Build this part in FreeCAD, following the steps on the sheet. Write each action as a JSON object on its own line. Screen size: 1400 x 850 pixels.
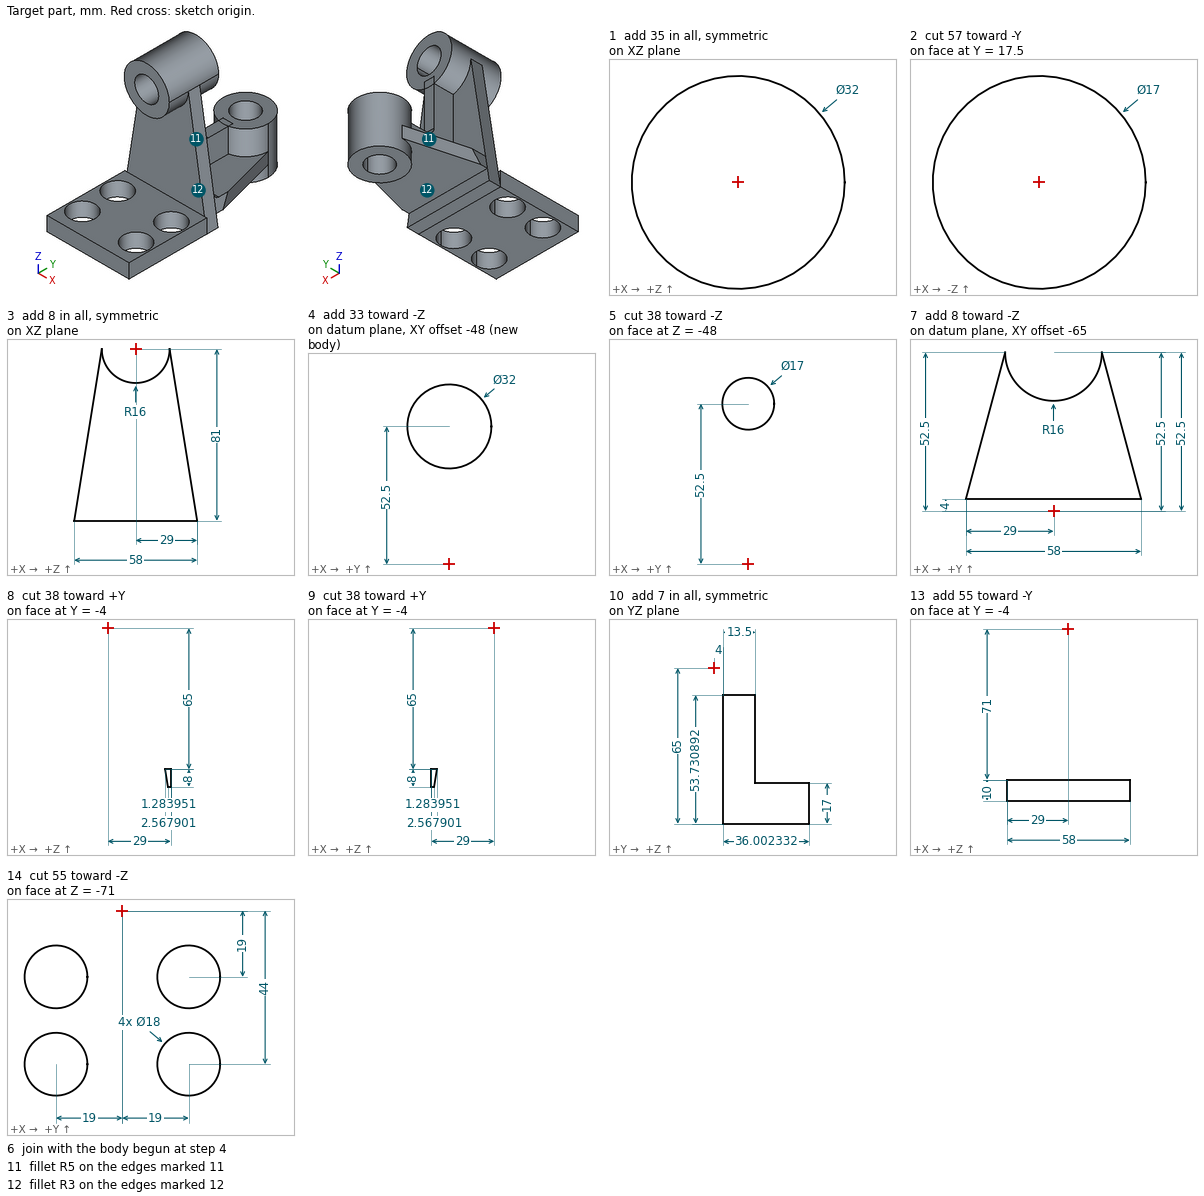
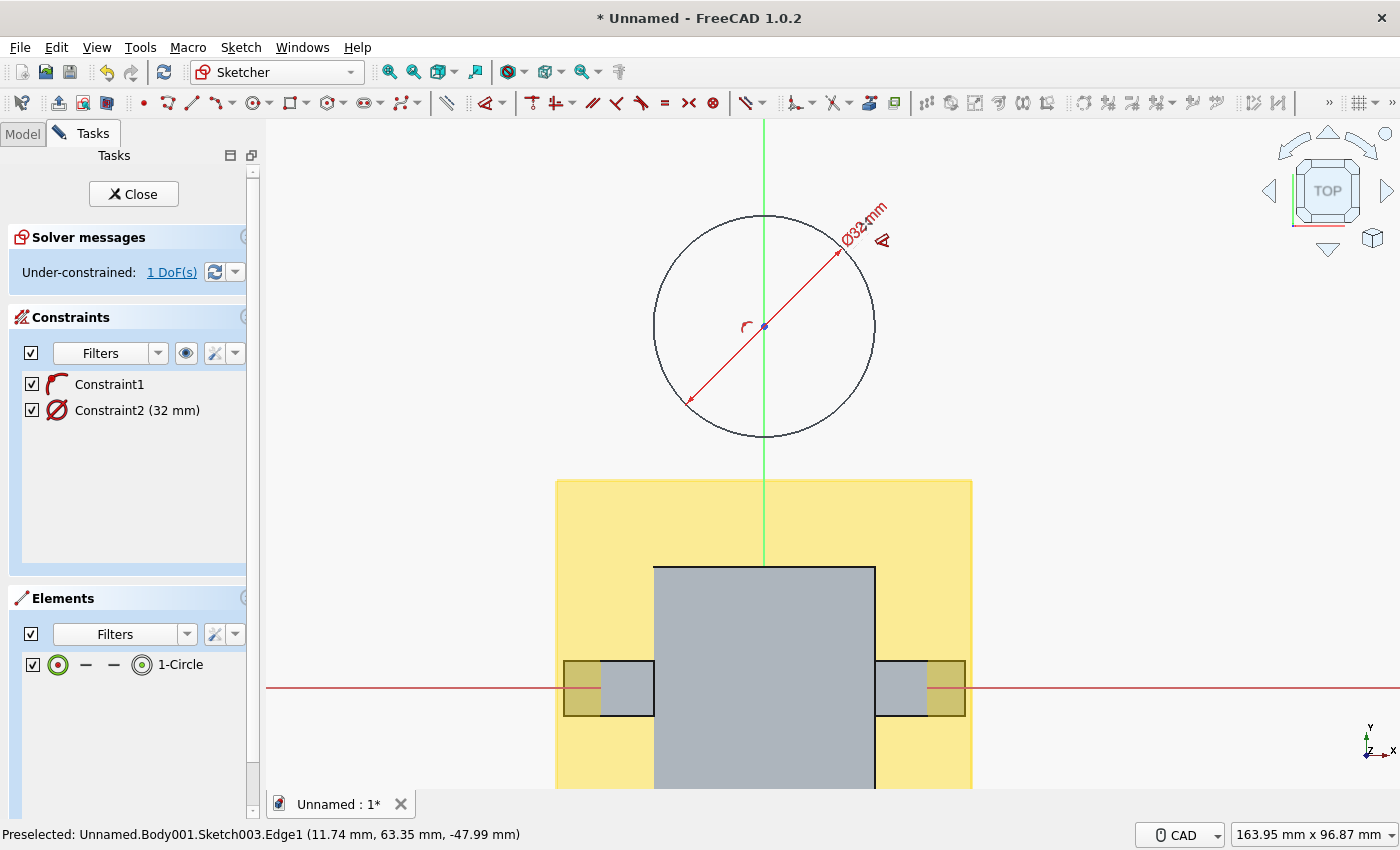
{"action": "left_click", "coordinate": [764, 326]}
{"action": "left_click", "coordinate": [798, 507]}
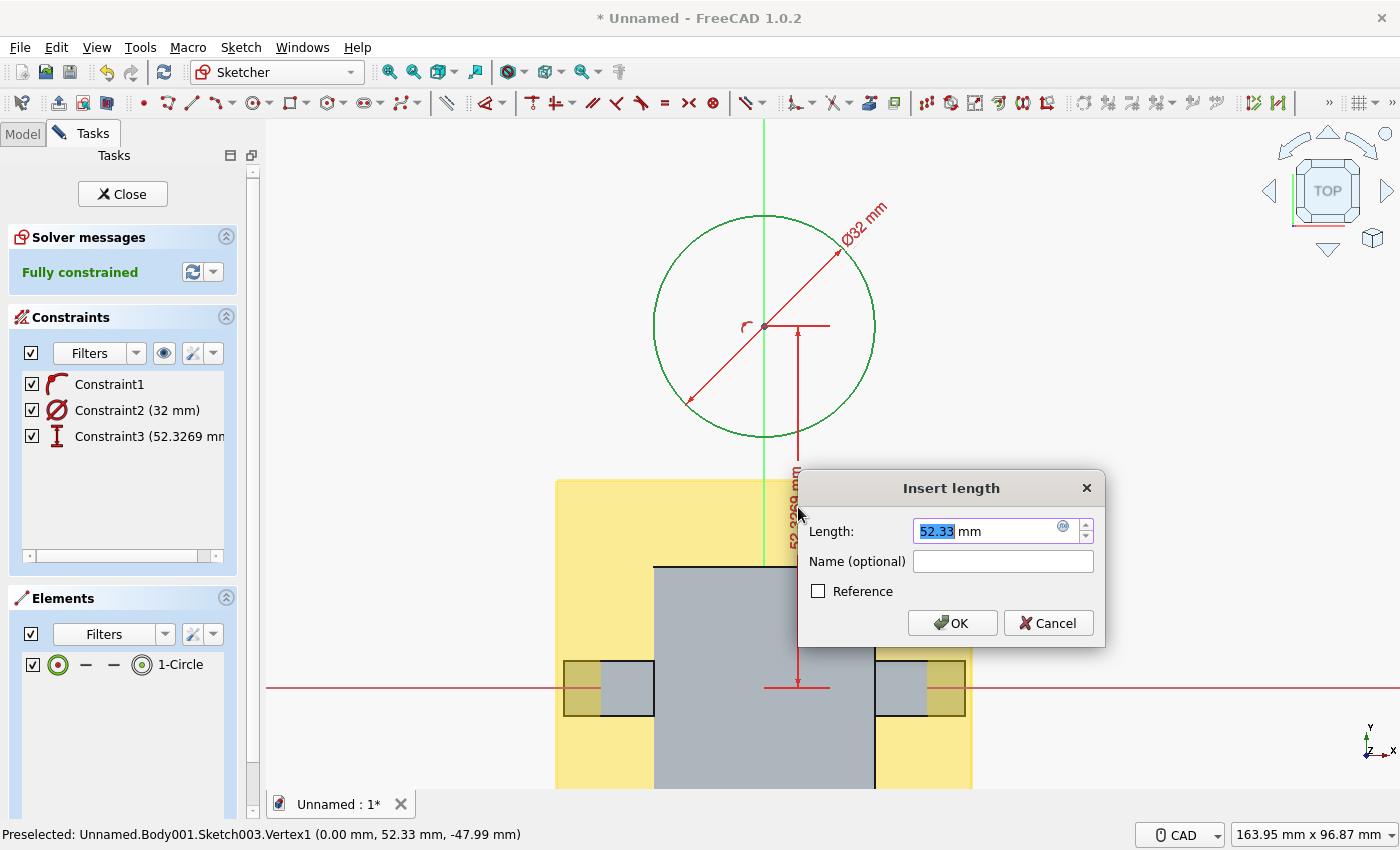
{"action": "type", "text": "52.5"}
{"action": "key", "text": "Return"}
{"action": "key", "text": "Escape"}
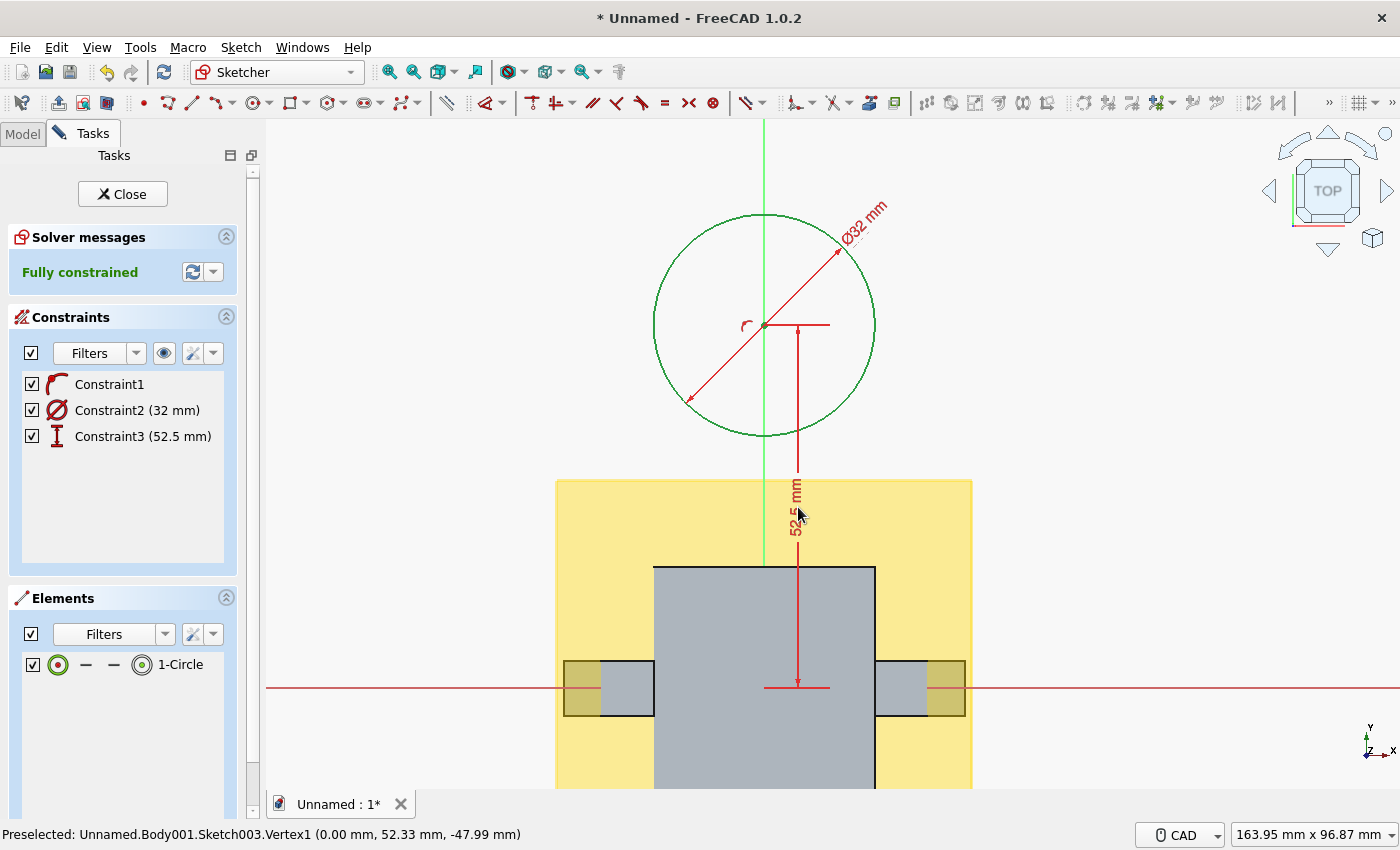
{"action": "left_click", "coordinate": [123, 194]}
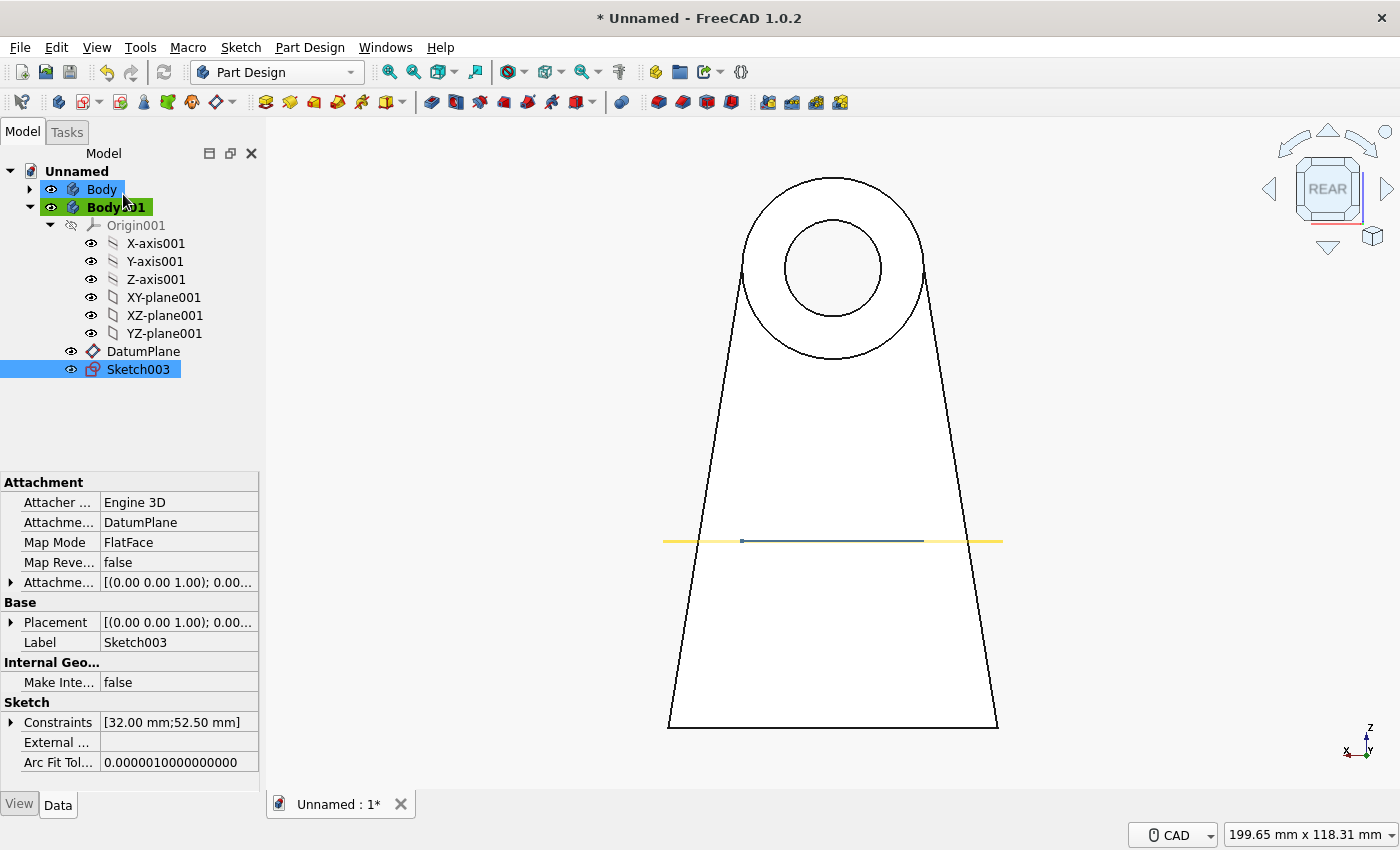
{"action": "left_click", "coordinate": [266, 102]}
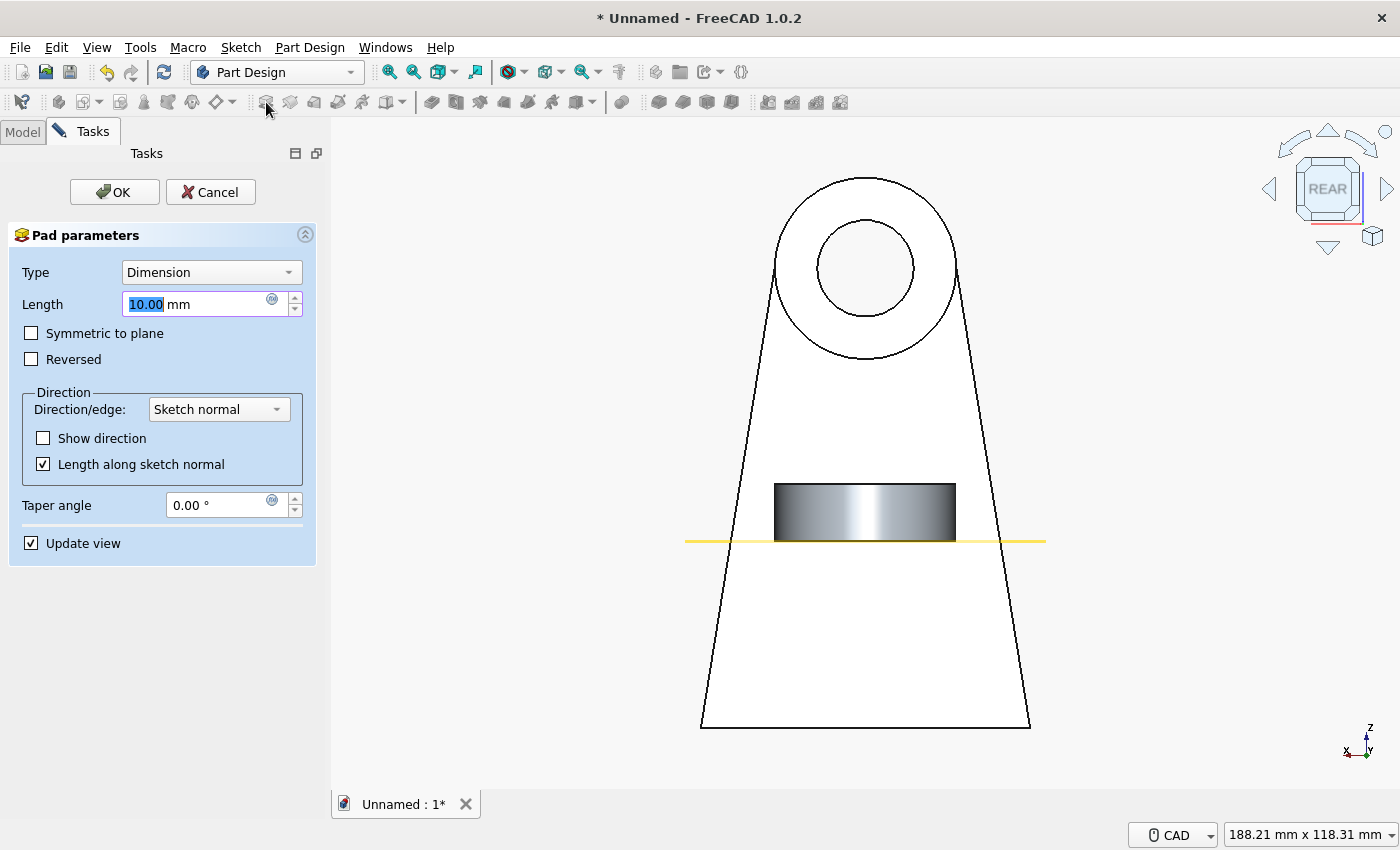
{"action": "type", "text": "33"}
{"action": "key", "text": "Tab"}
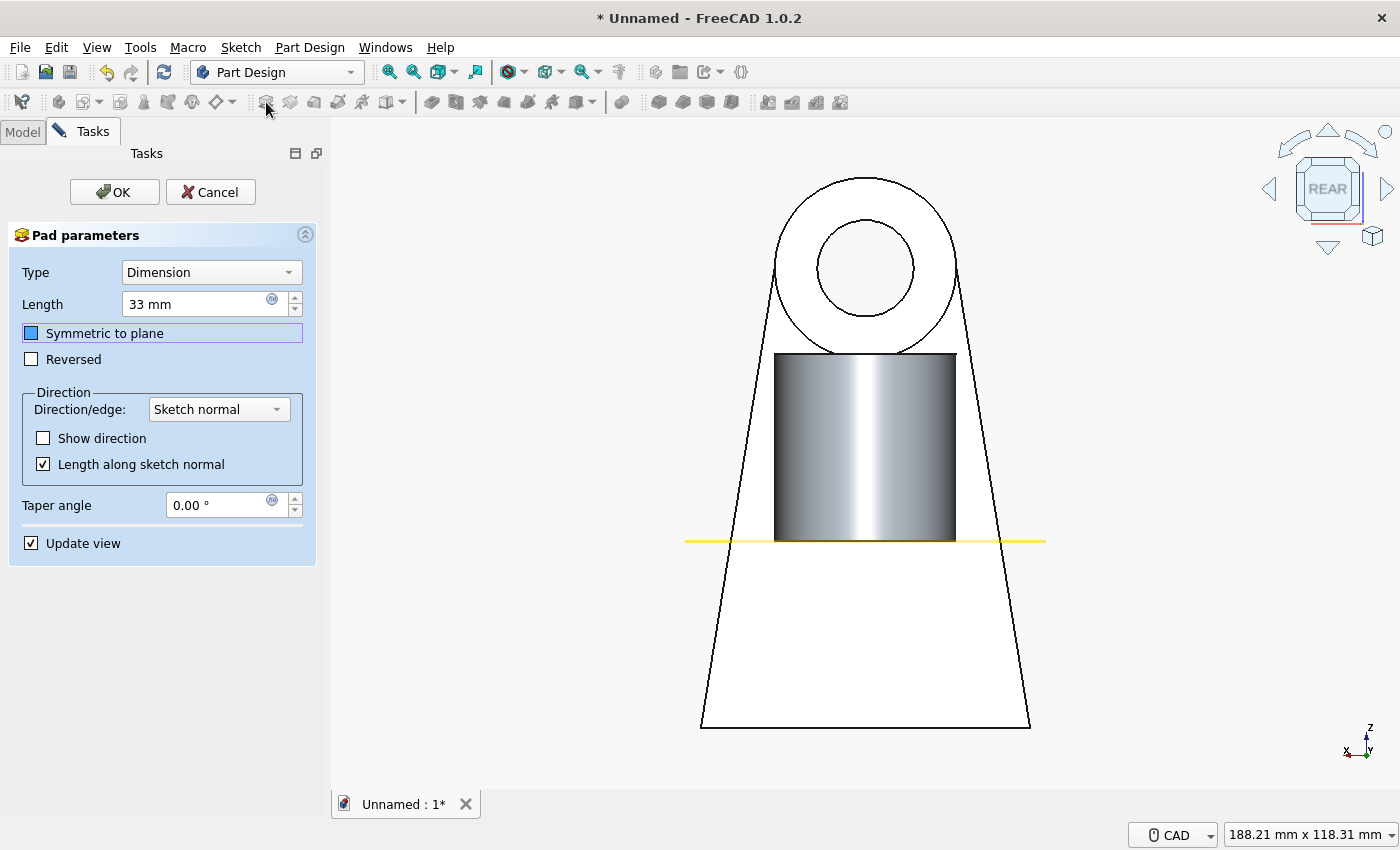
{"action": "left_click", "coordinate": [30, 359]}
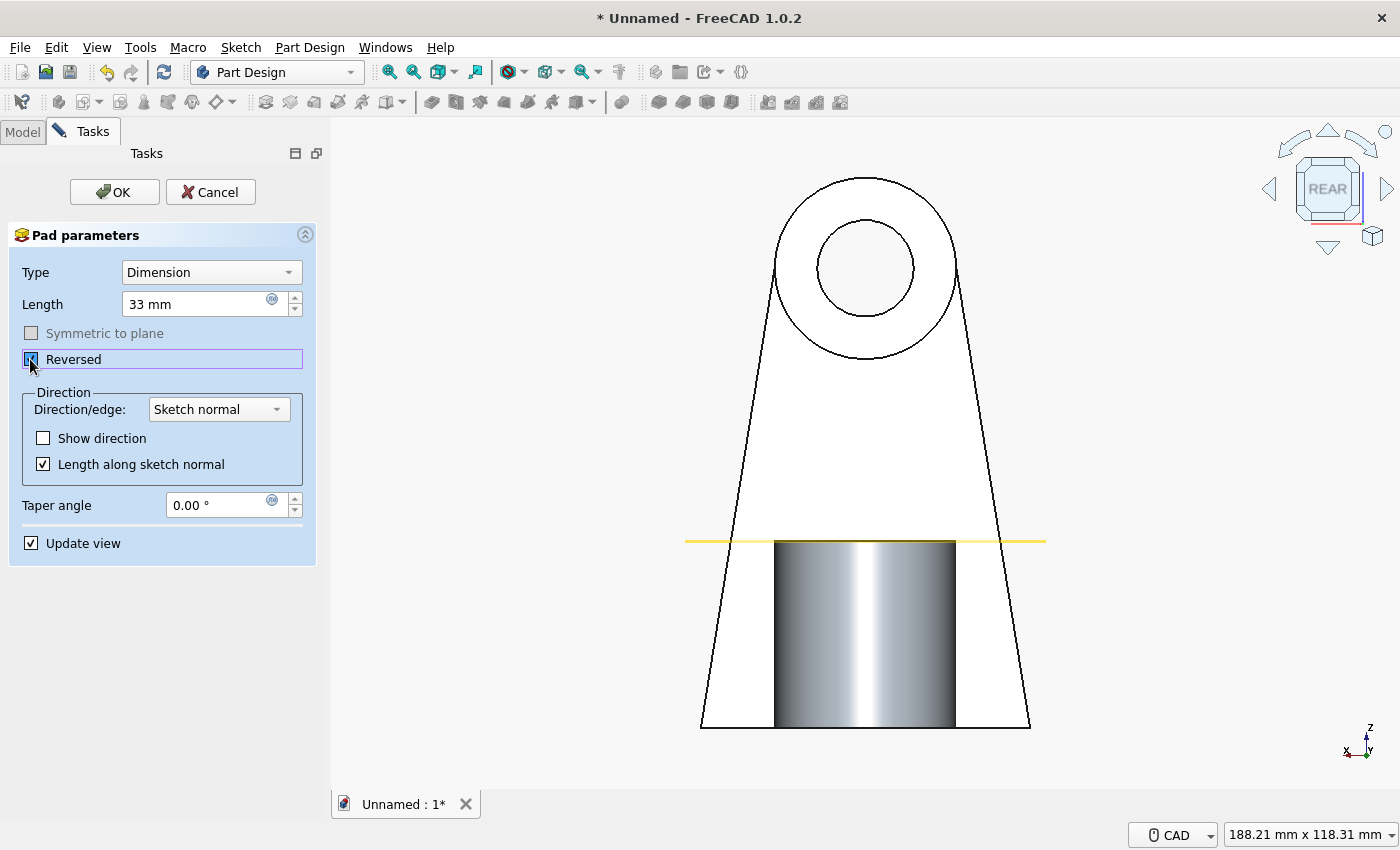
{"action": "left_click", "coordinate": [115, 192]}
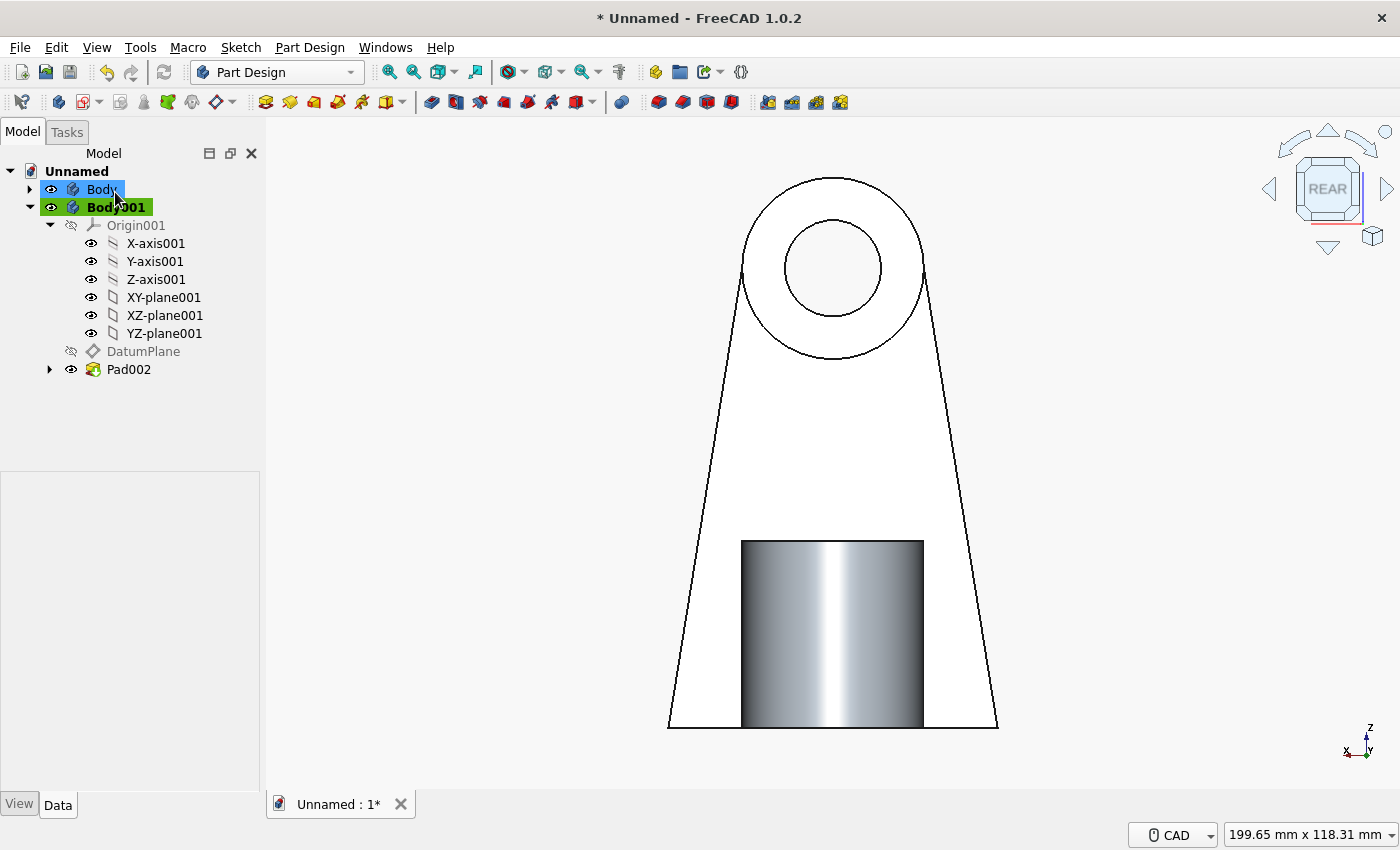
{"action": "left_click", "coordinate": [390, 72]}